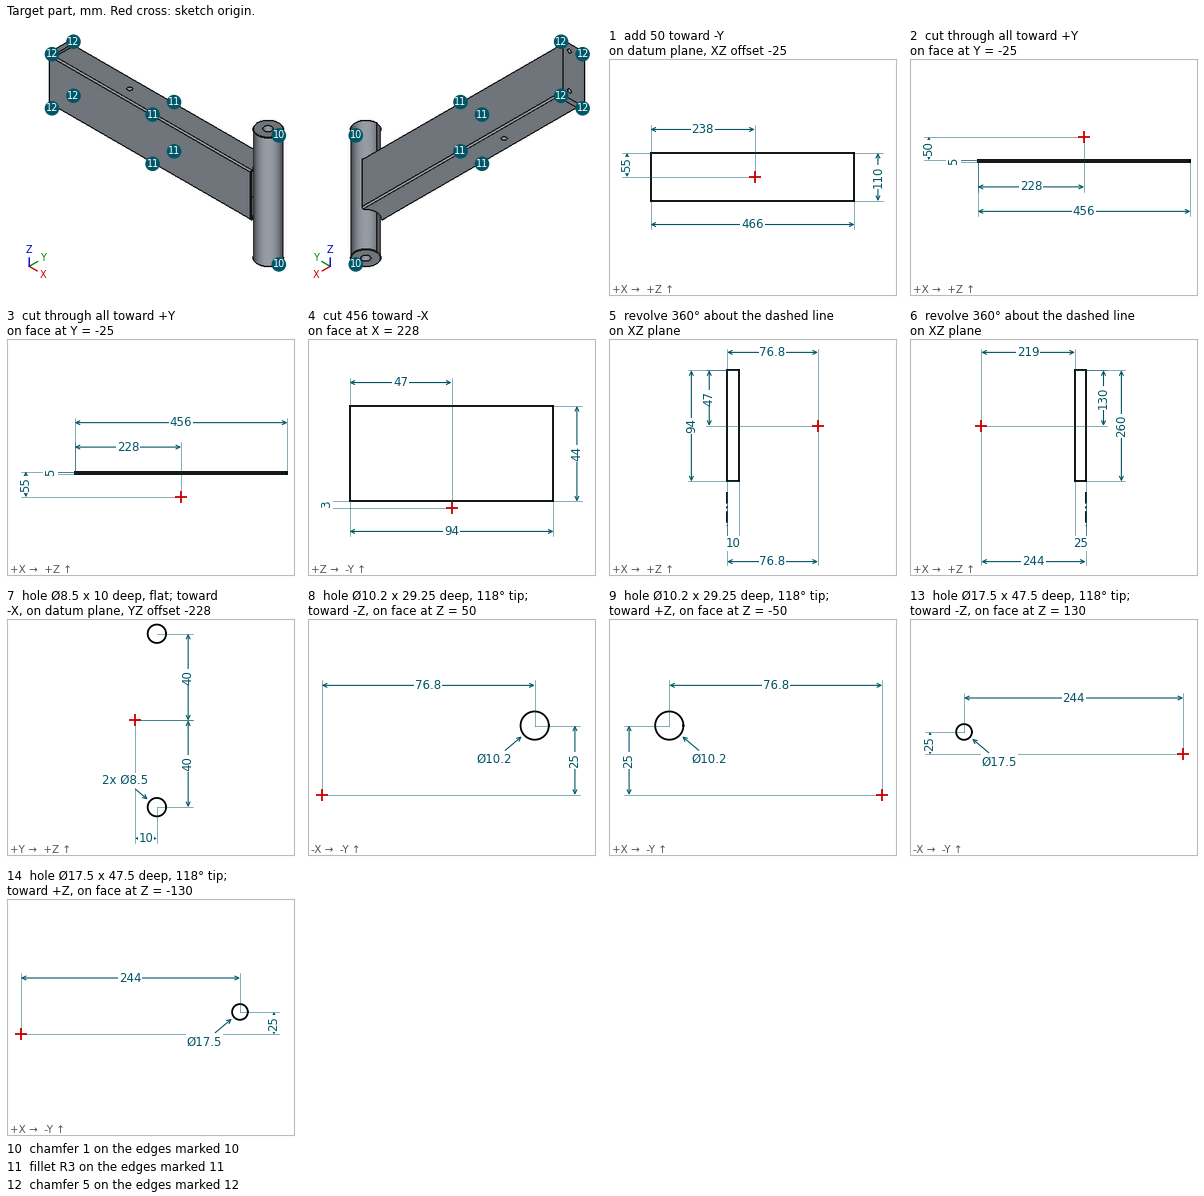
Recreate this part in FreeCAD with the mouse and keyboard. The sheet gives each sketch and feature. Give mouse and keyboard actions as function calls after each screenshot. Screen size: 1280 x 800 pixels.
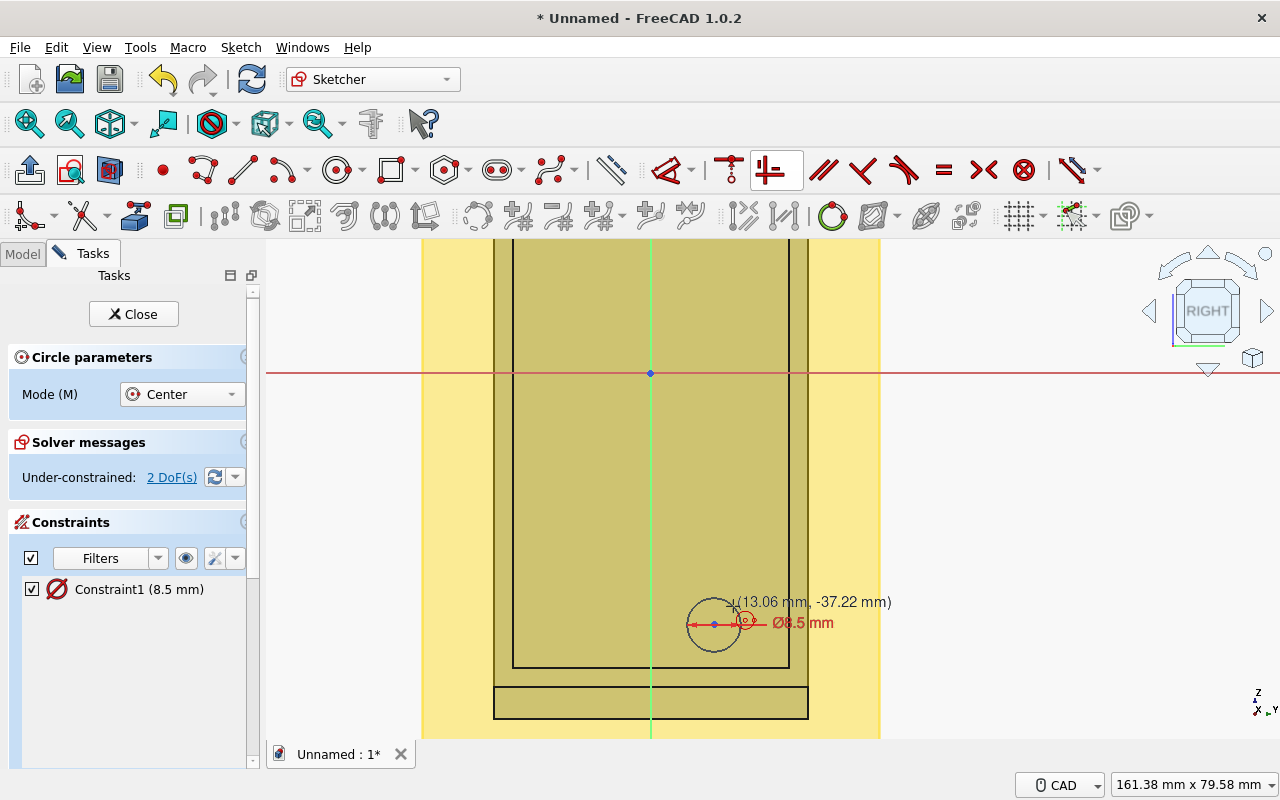
scroll(715, 630, down, 3)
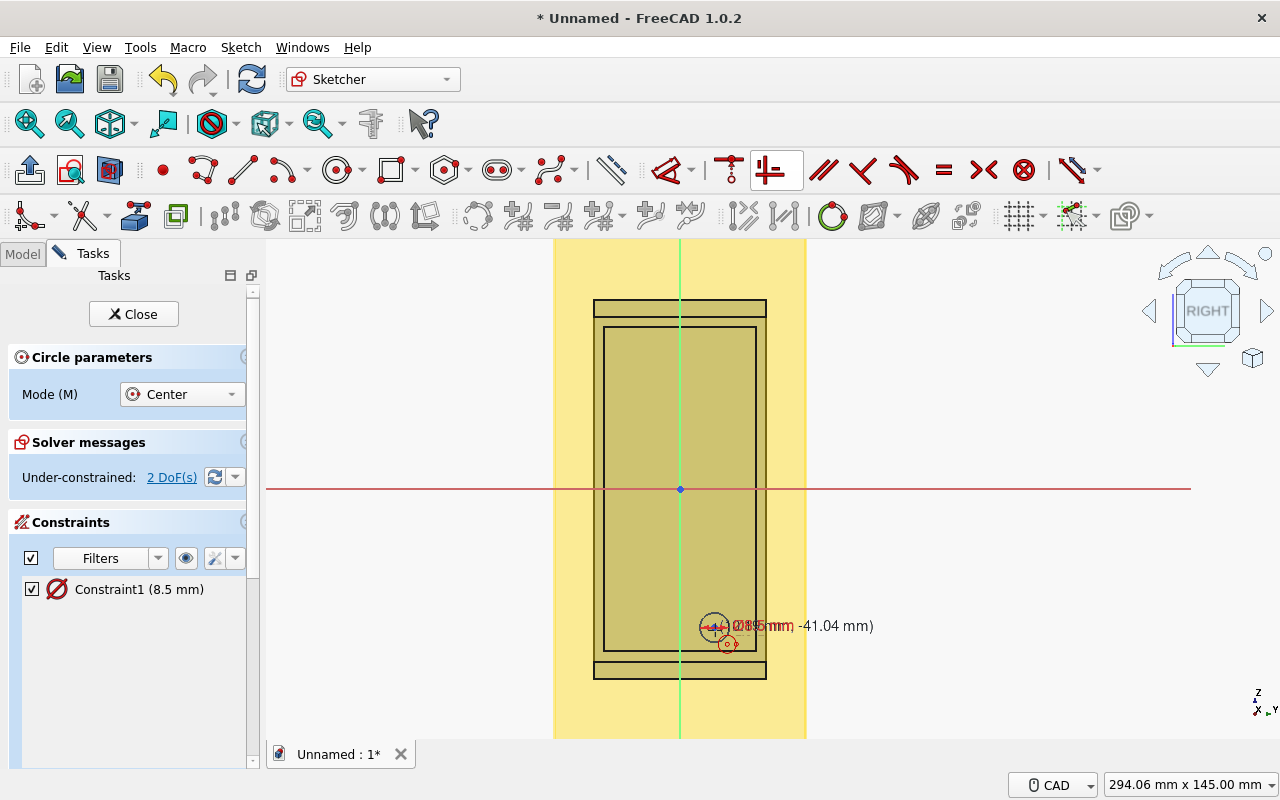
scroll(715, 351, up, 3)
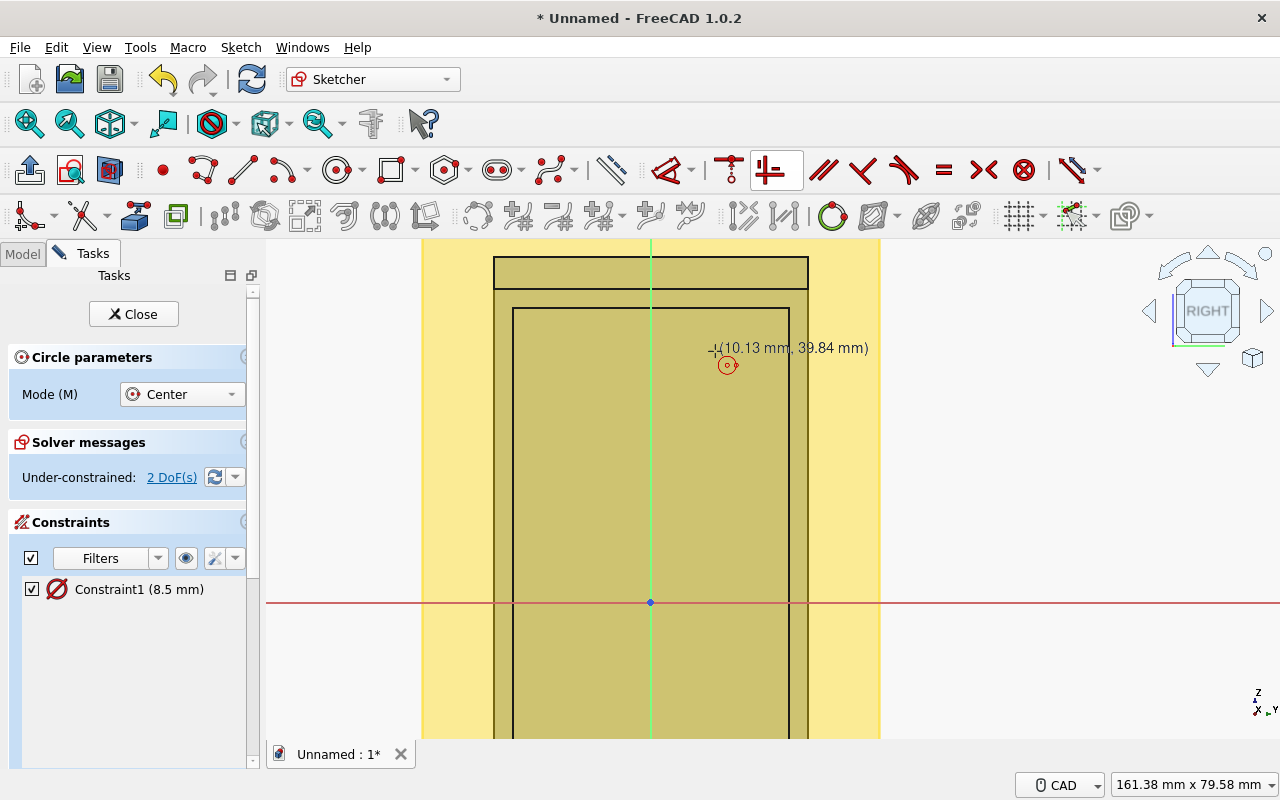
click(714, 352)
move(733, 333)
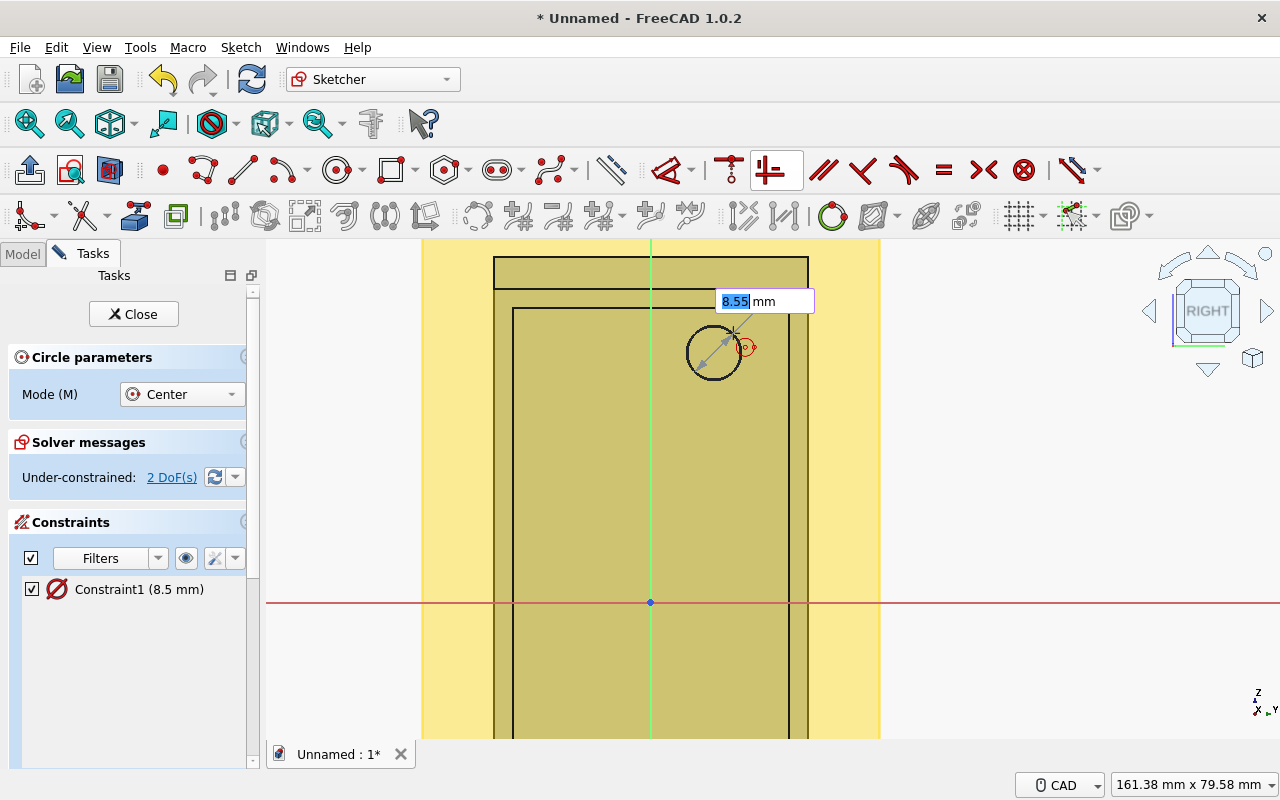
text(8.5)
key(Return)
key(Escape)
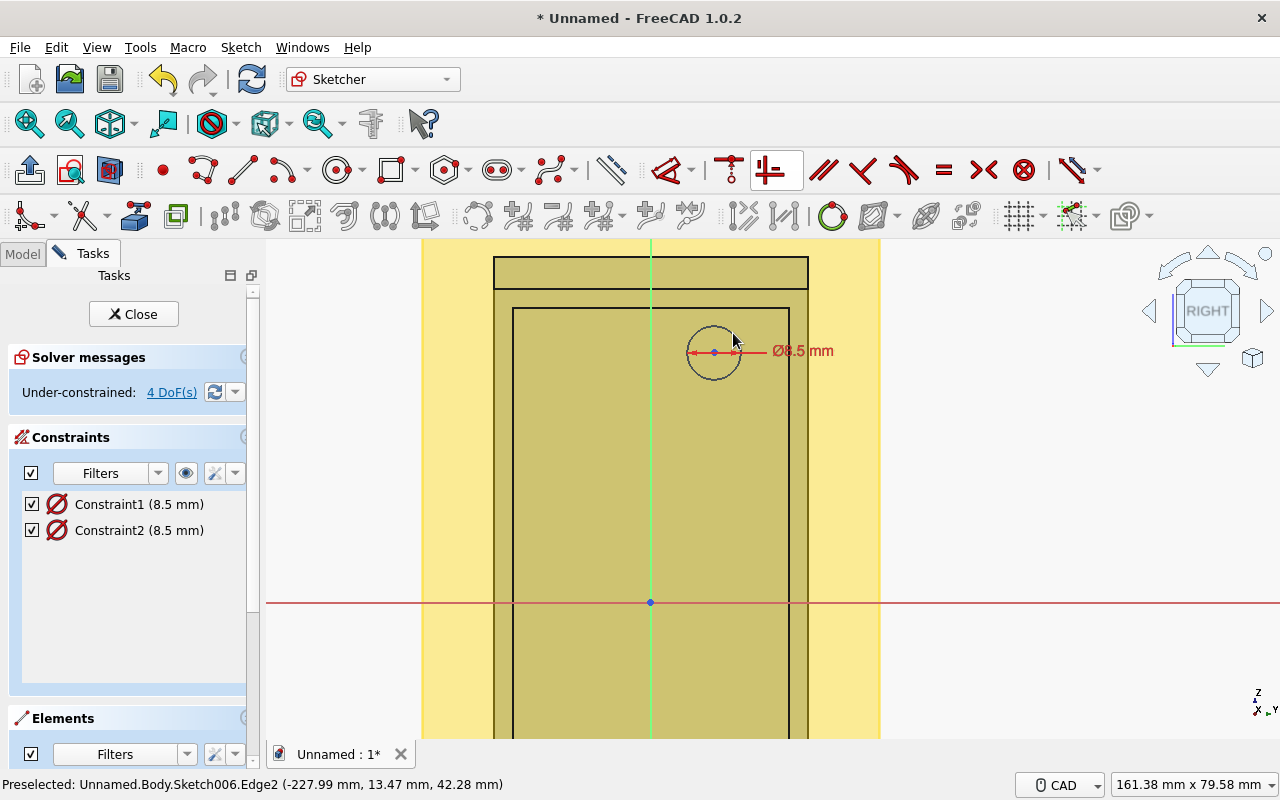
scroll(715, 350, down, 3)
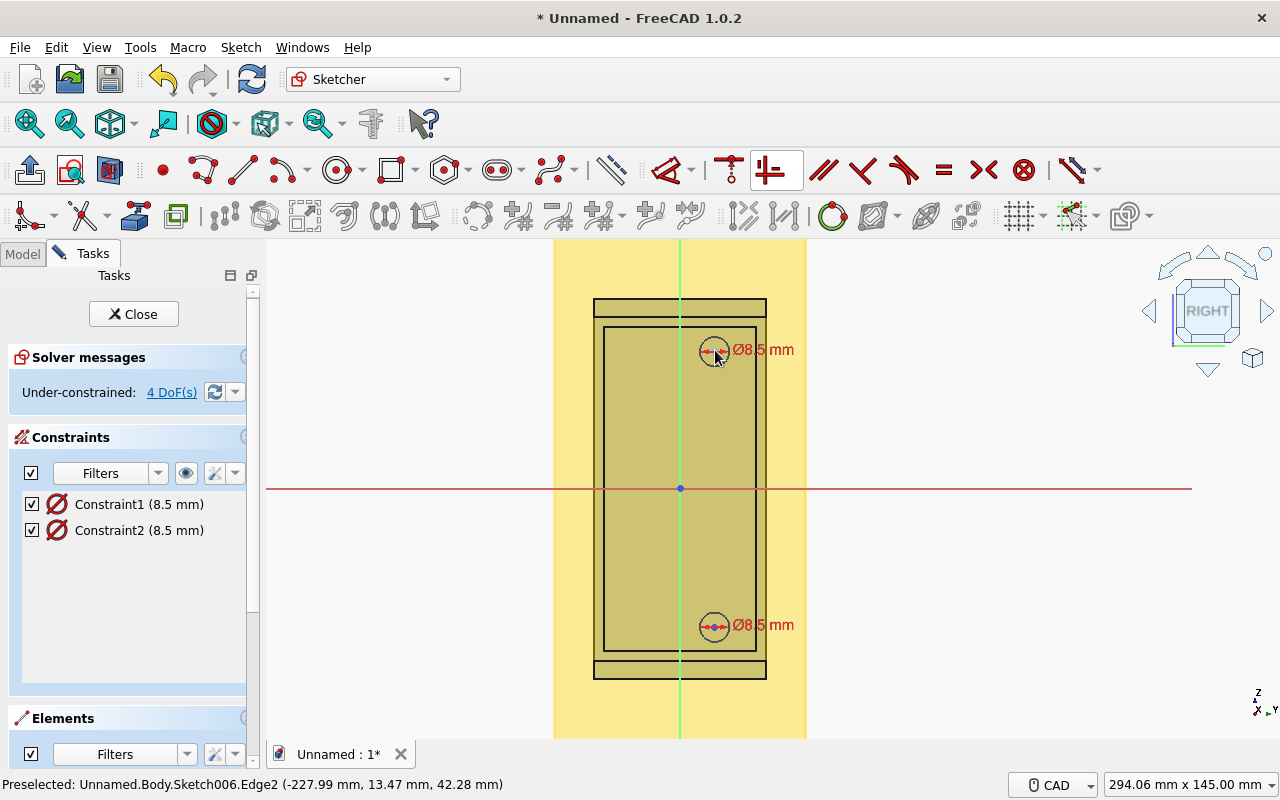
click(715, 627)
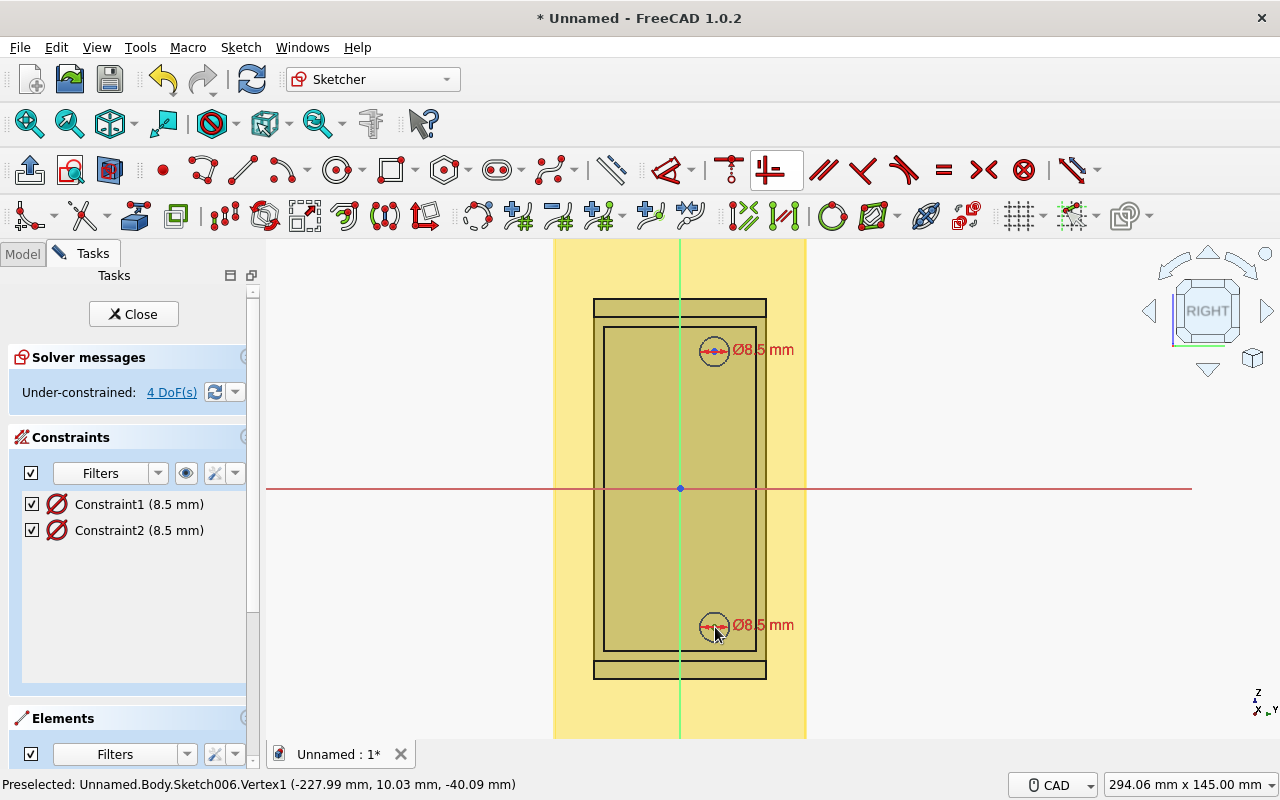
click(715, 352)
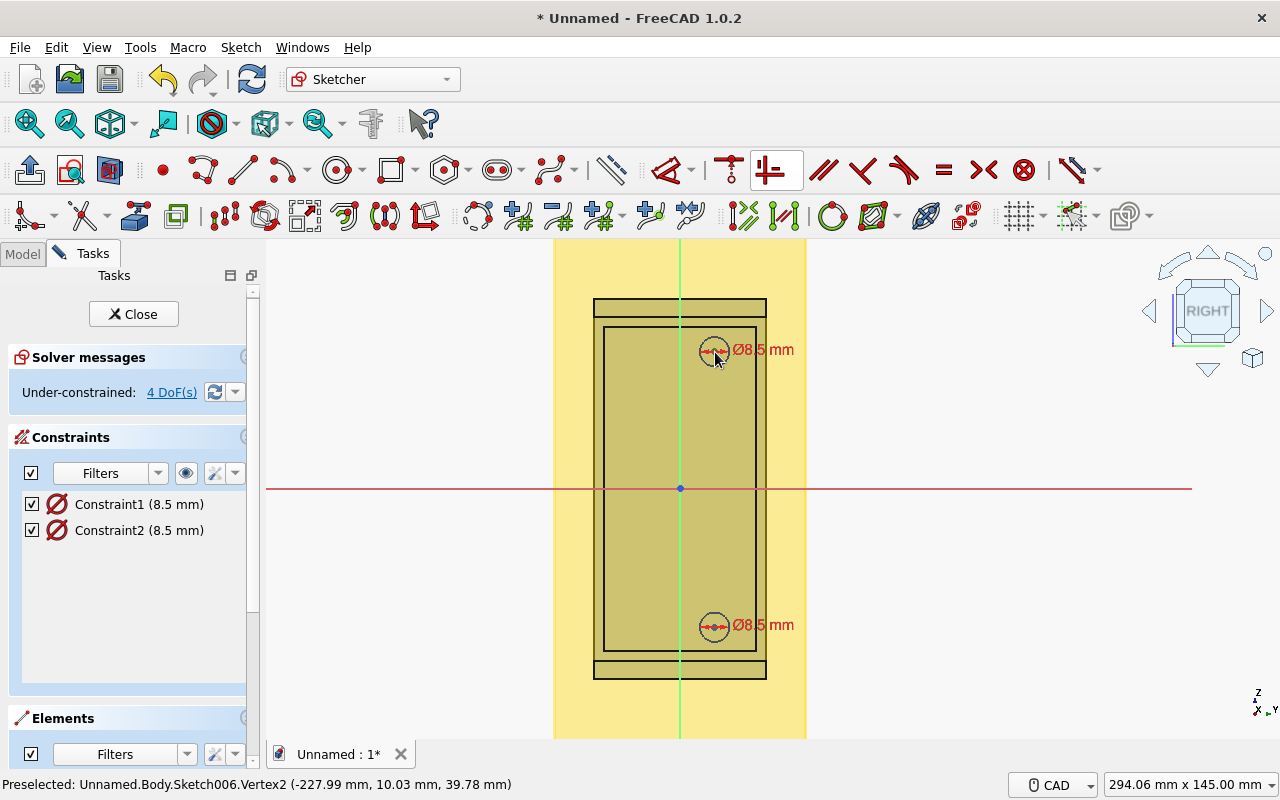
click(798, 170)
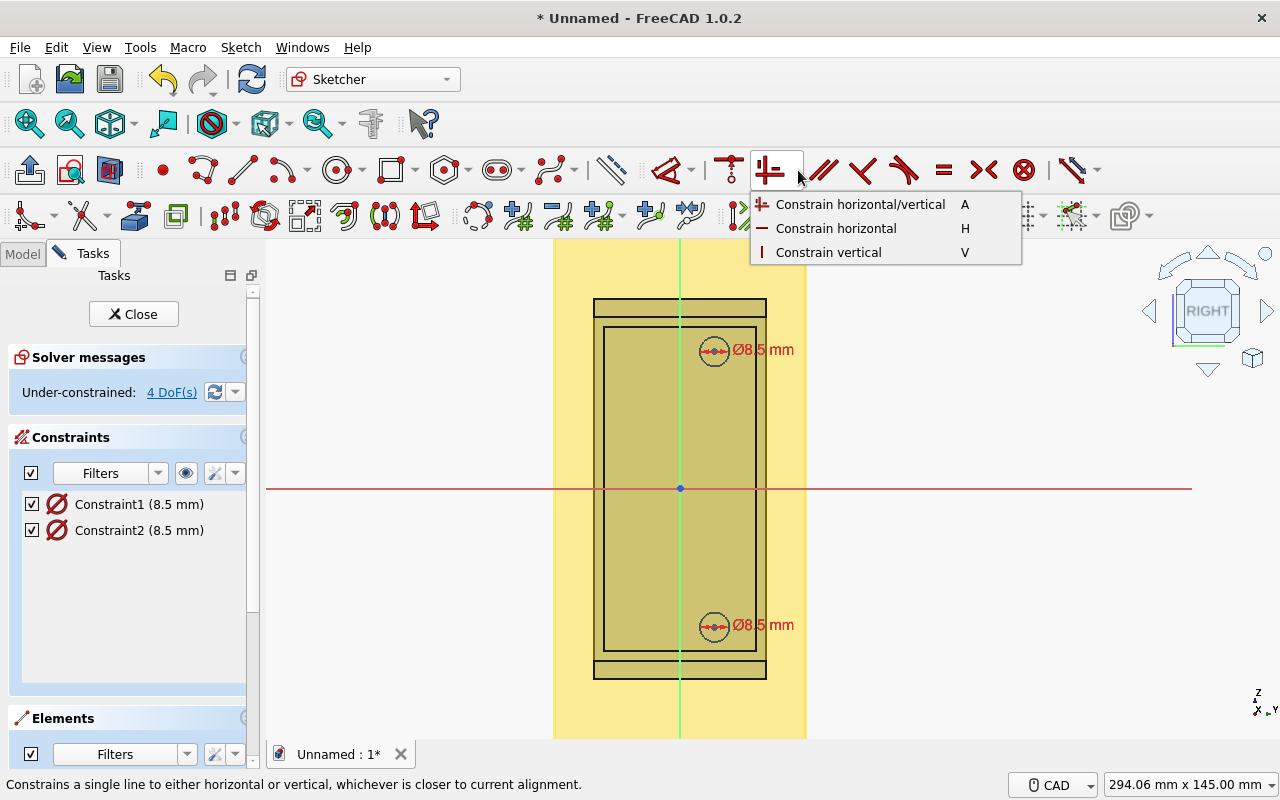
click(886, 252)